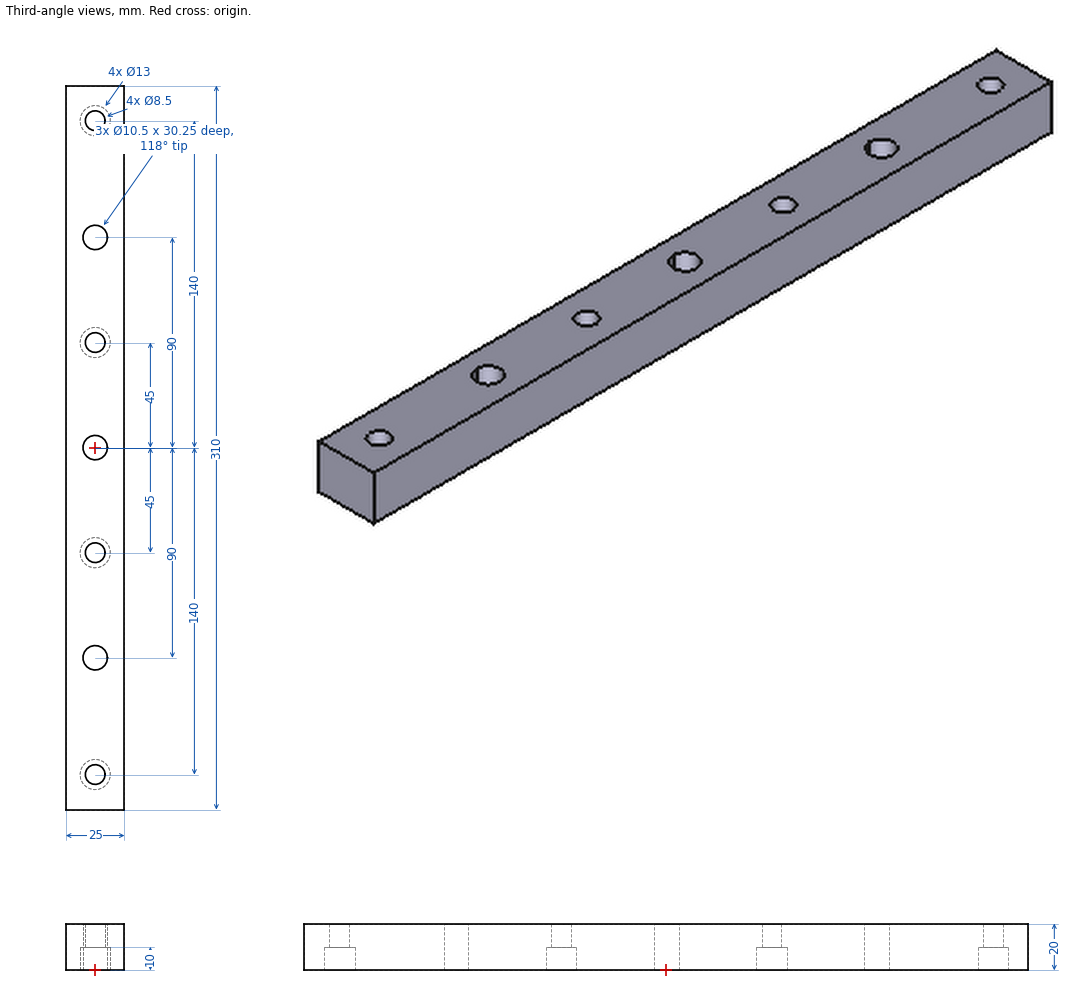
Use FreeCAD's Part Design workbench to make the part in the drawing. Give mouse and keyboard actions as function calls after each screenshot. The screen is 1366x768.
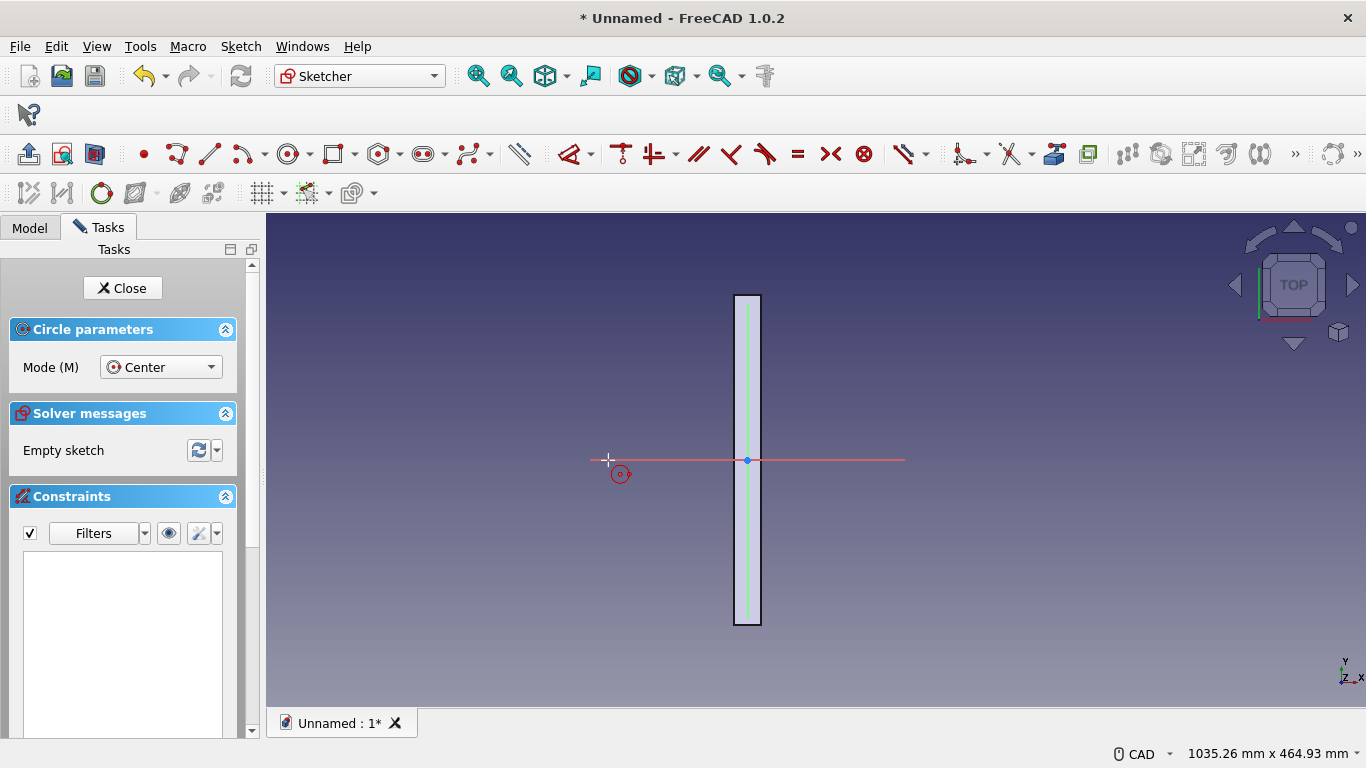
scroll(748, 311, up, 9)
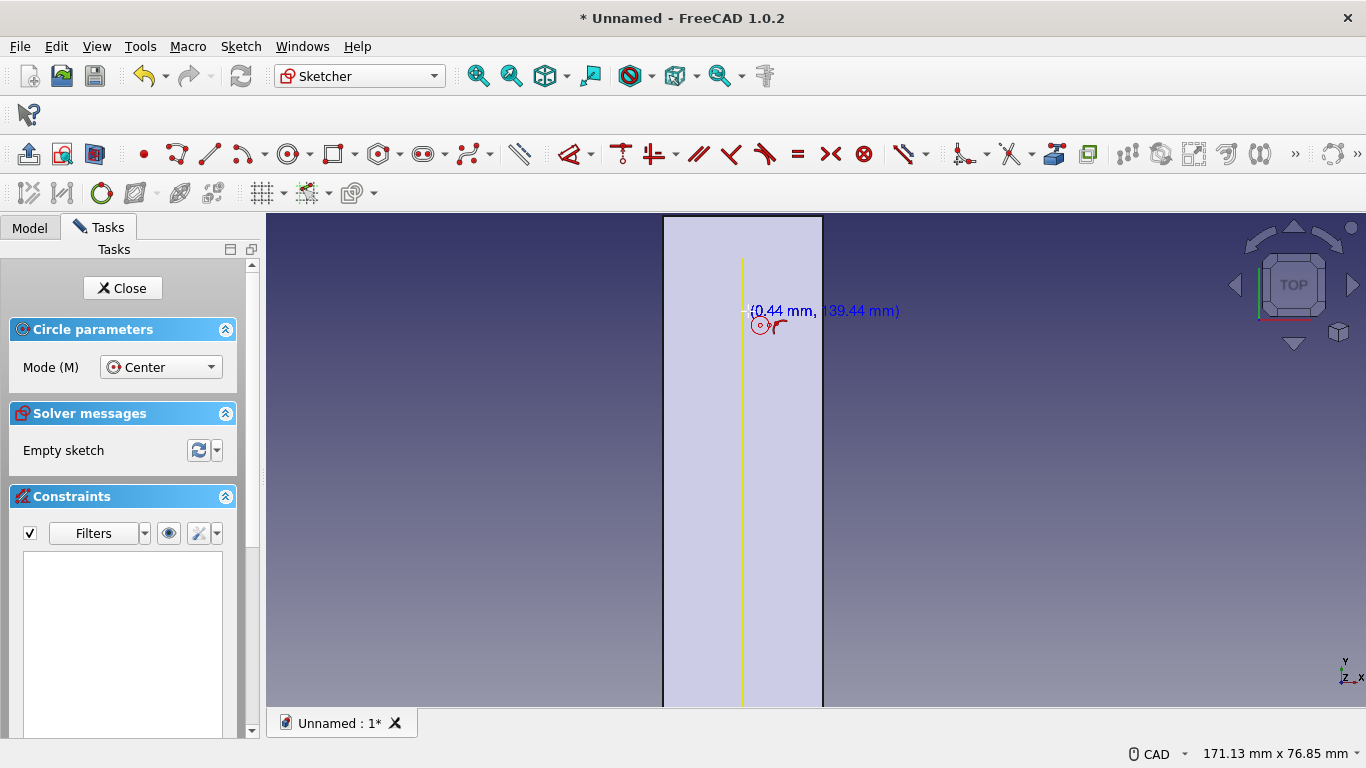
scroll(748, 311, down, 9)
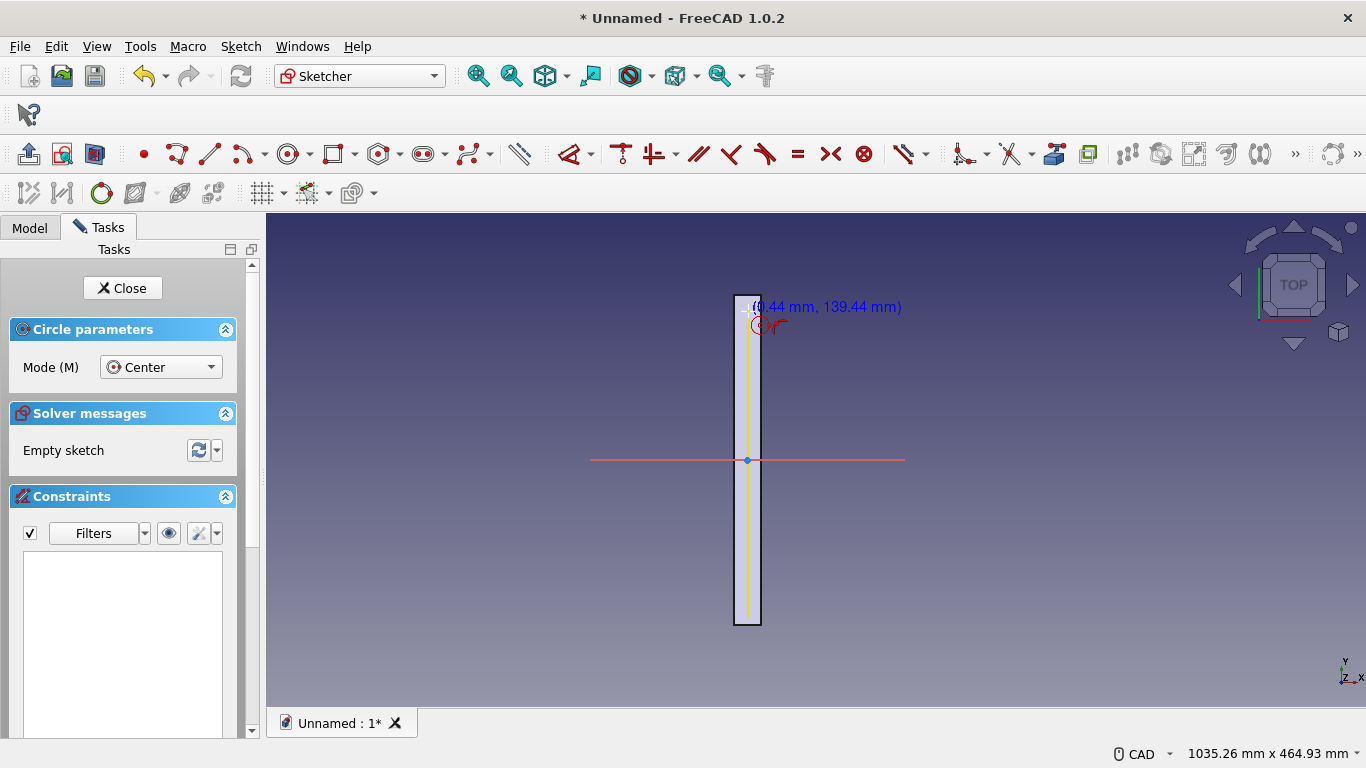
click(748, 311)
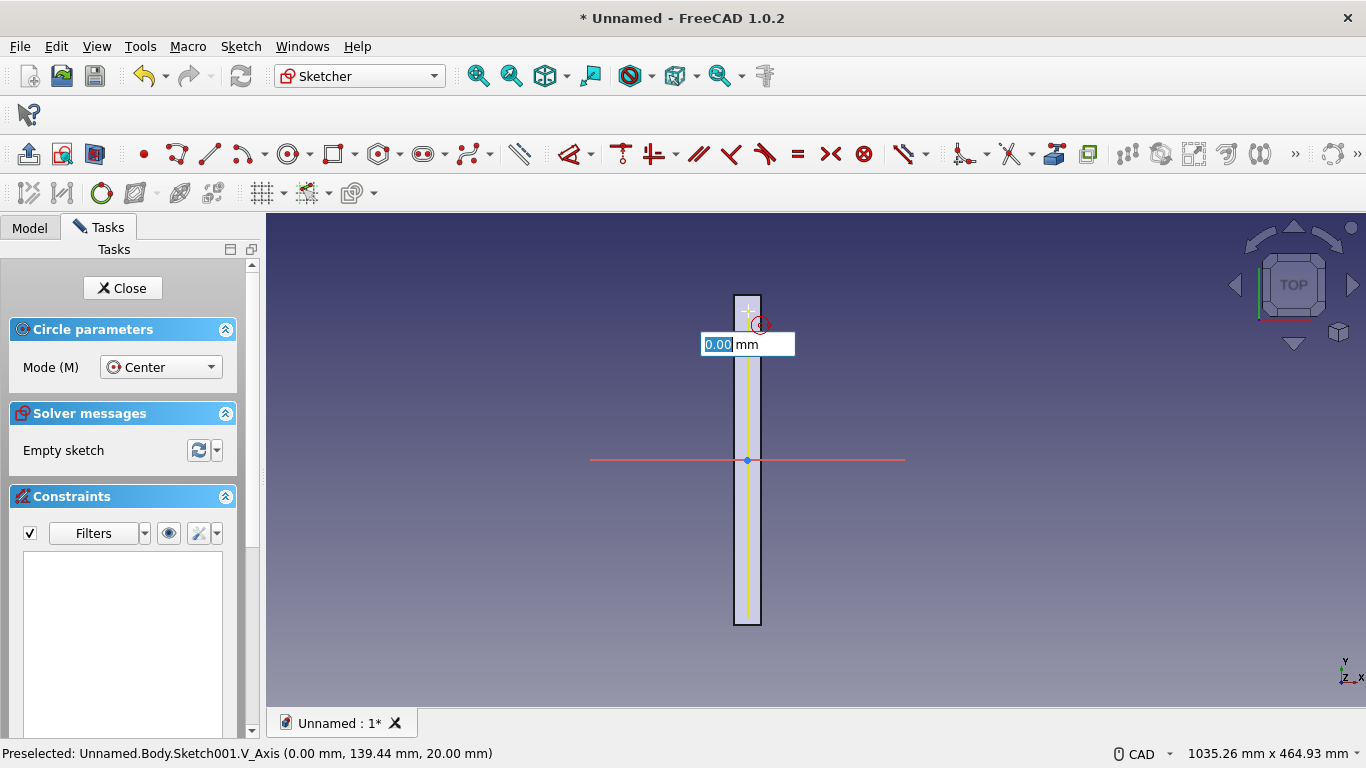
scroll(752, 310, up, 7)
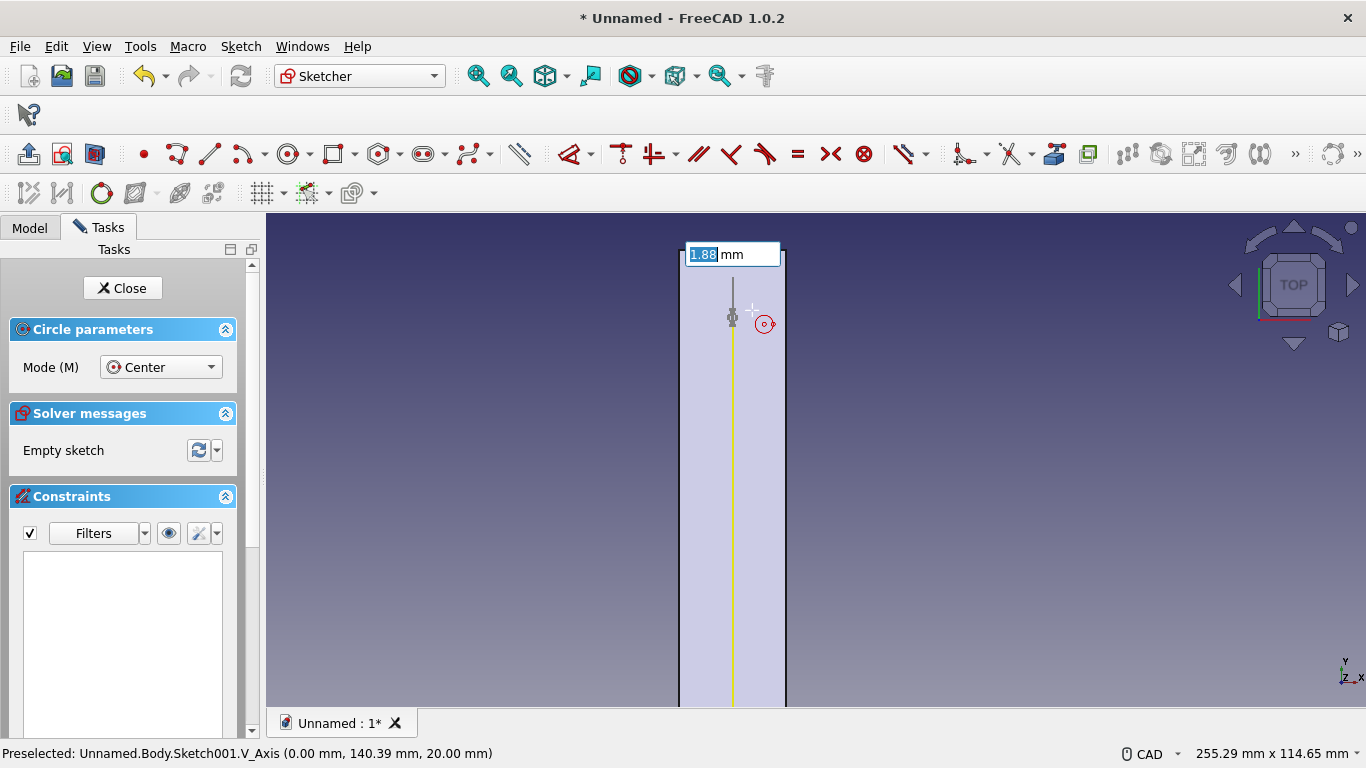
click(750, 309)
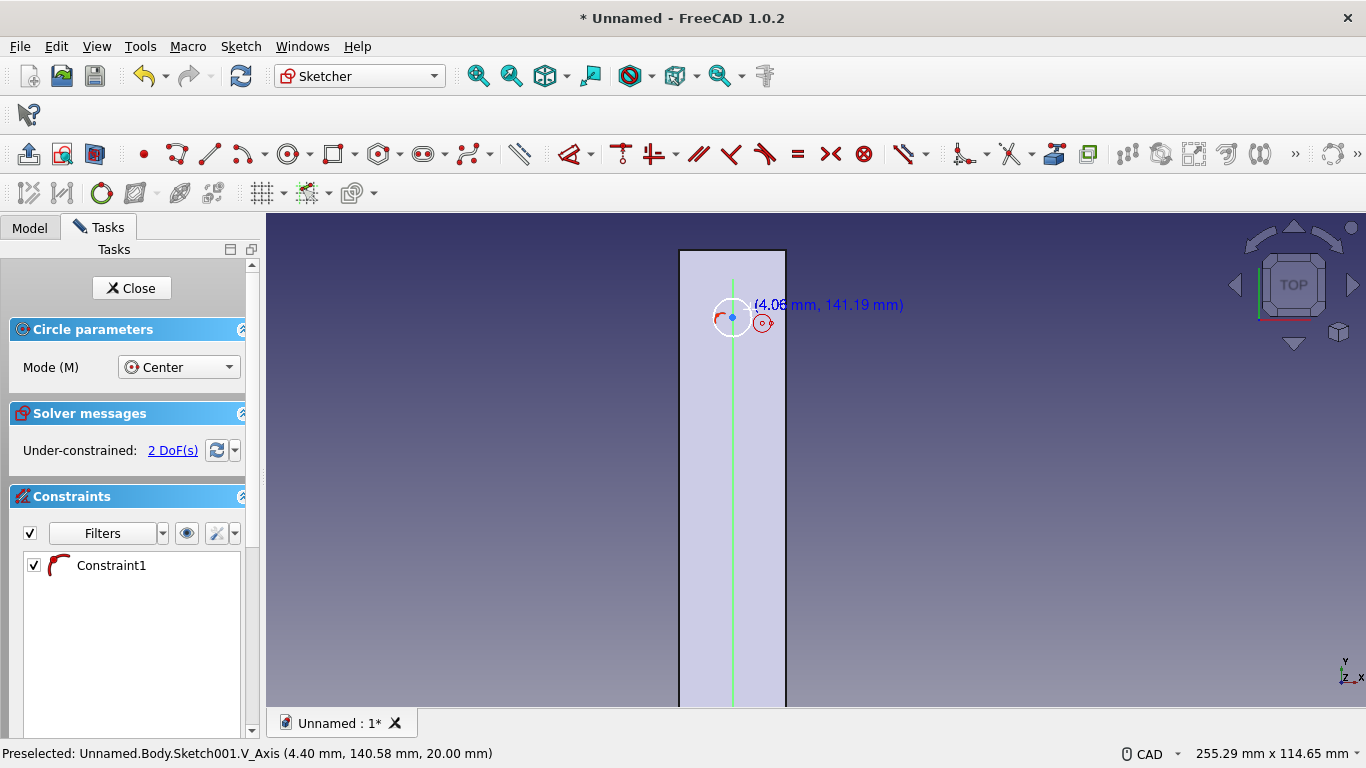
scroll(752, 310, down, 7)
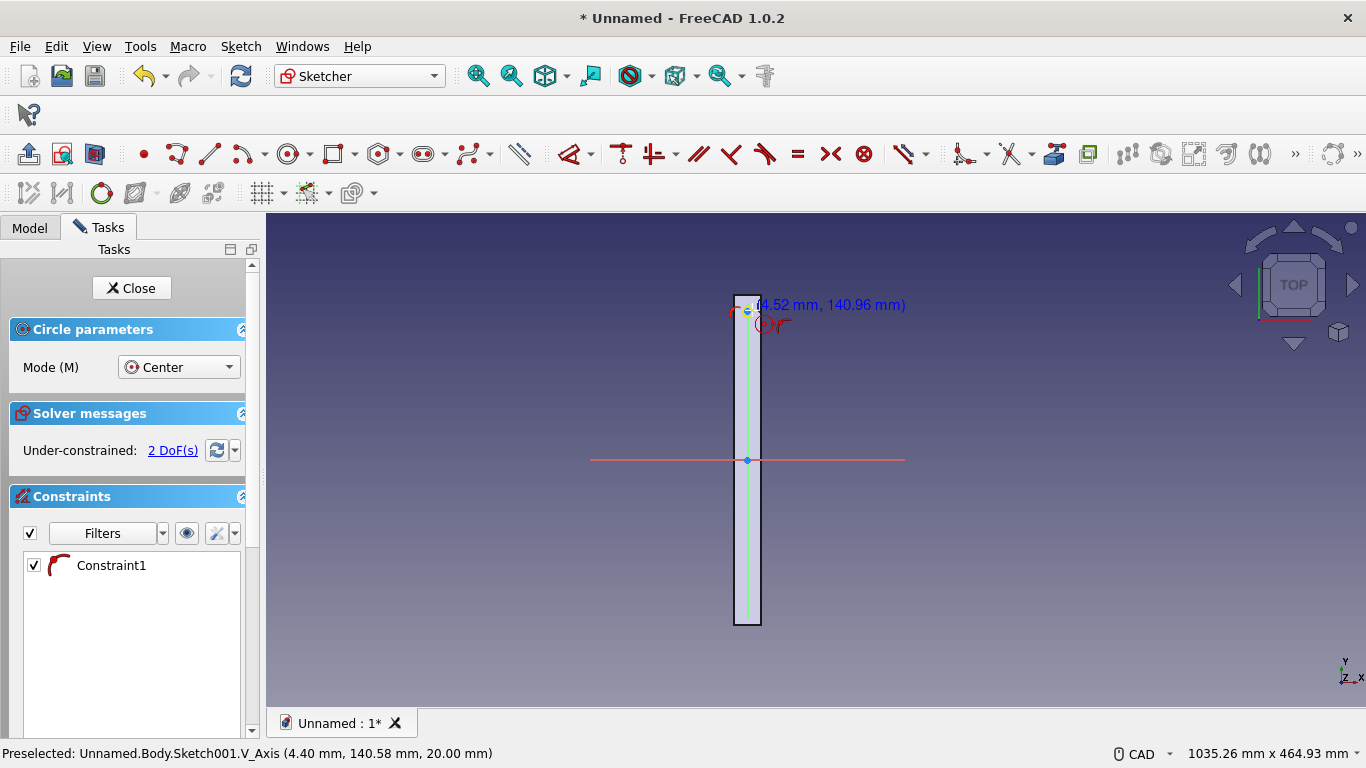
scroll(748, 412, up, 9)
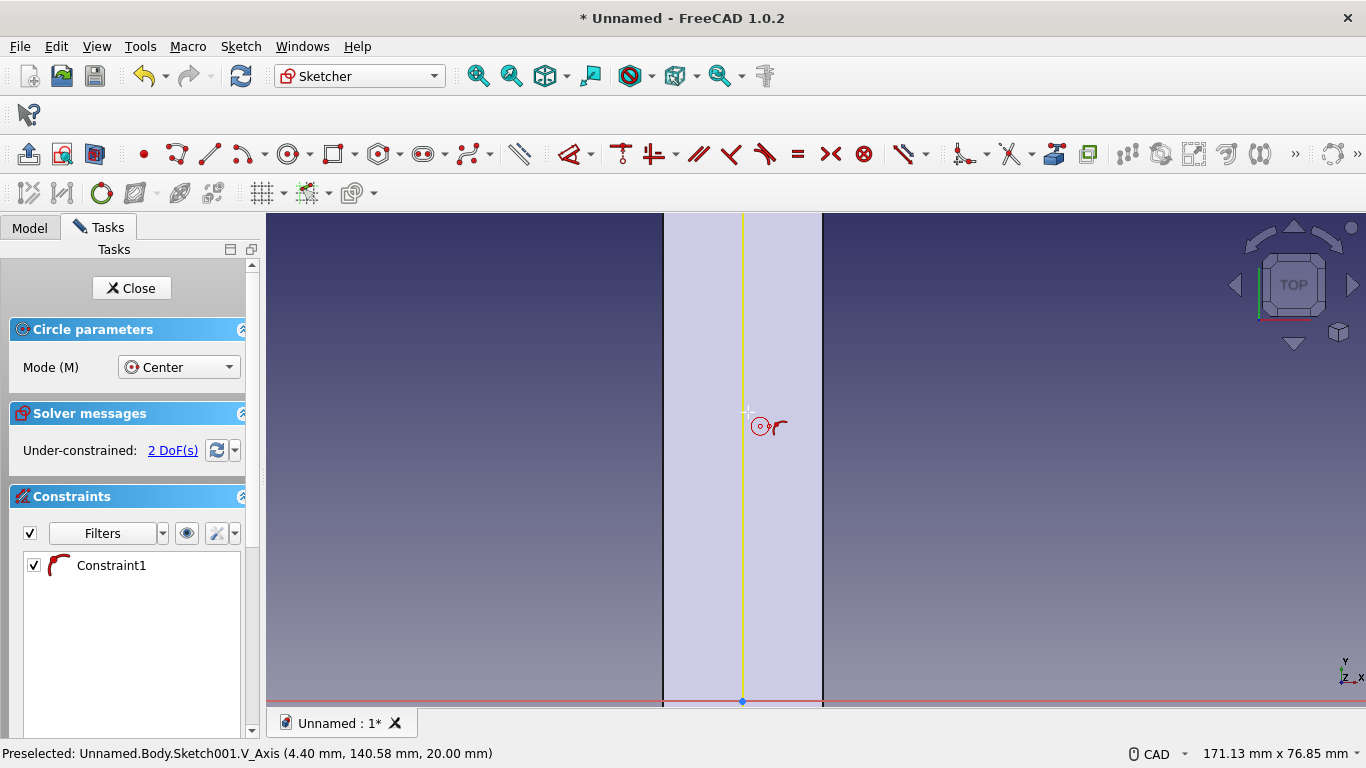
scroll(748, 412, down, 9)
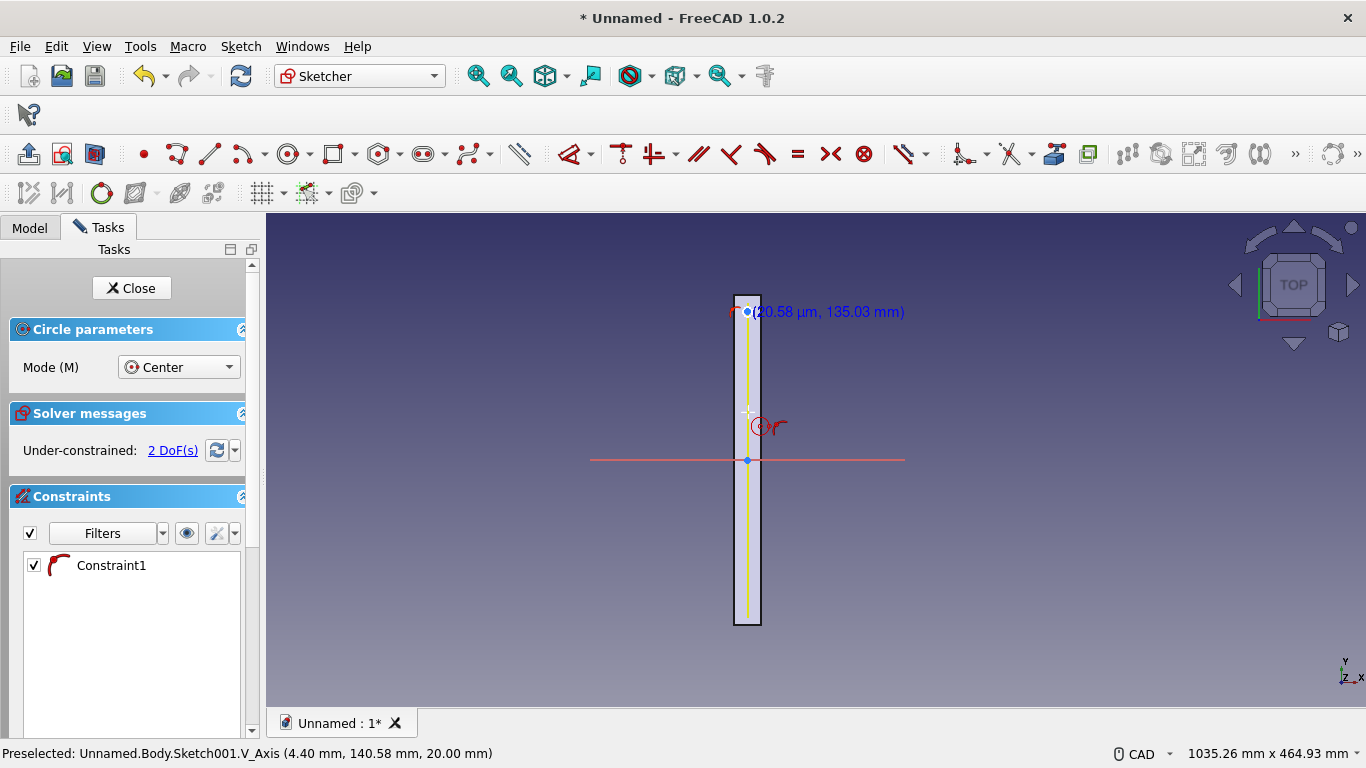
click(748, 412)